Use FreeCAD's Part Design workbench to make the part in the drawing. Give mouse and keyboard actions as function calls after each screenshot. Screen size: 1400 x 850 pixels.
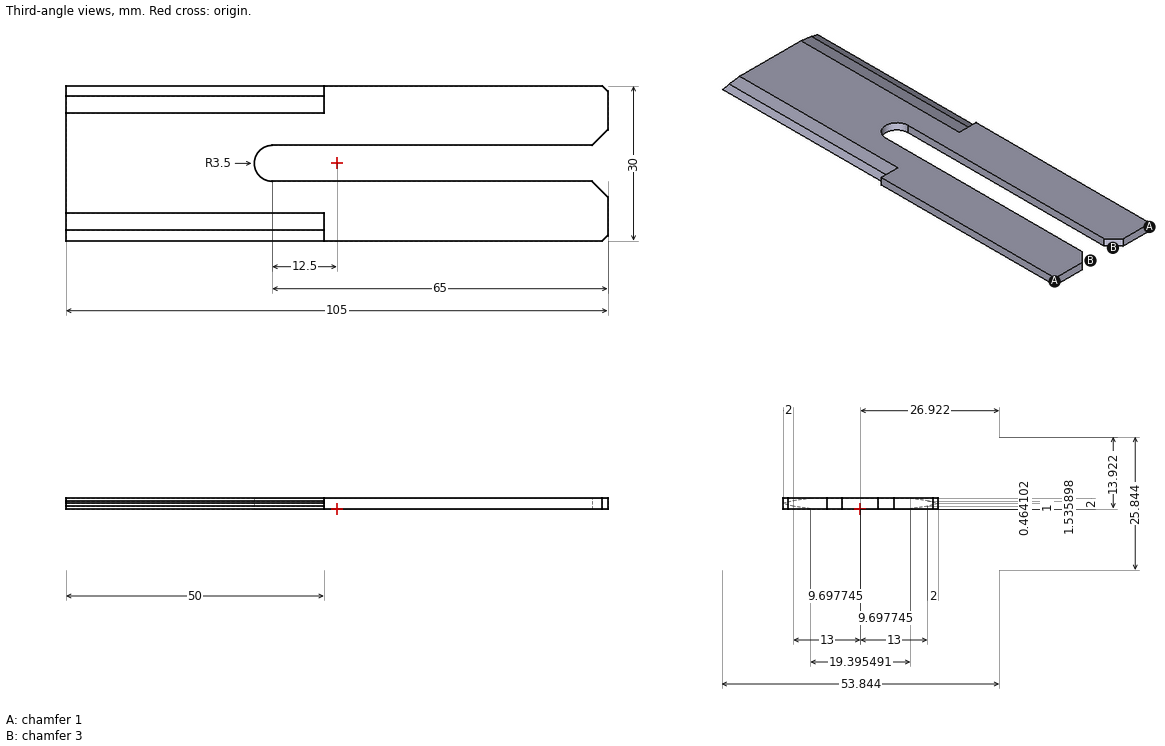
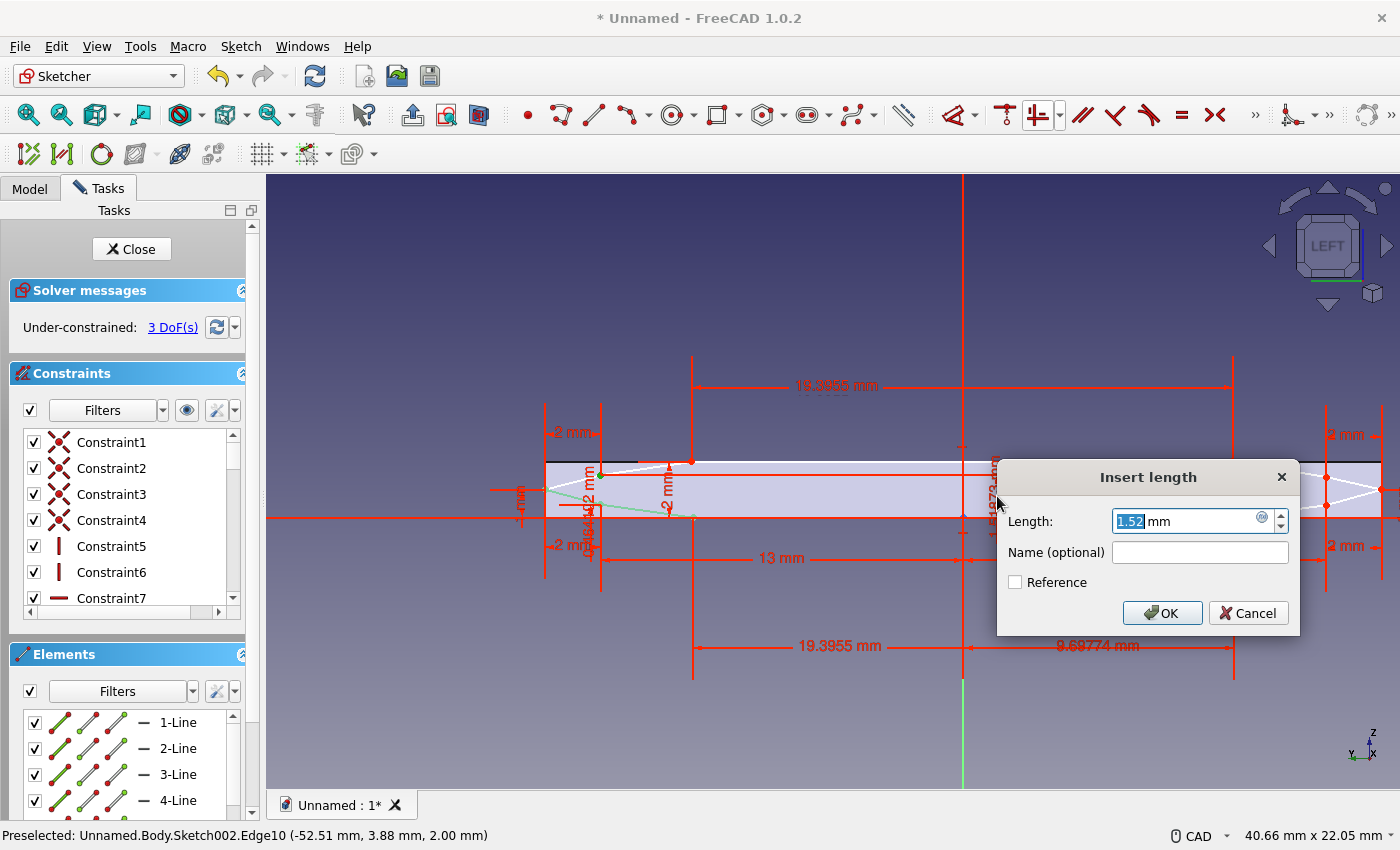
text(1.535898)
key(Return)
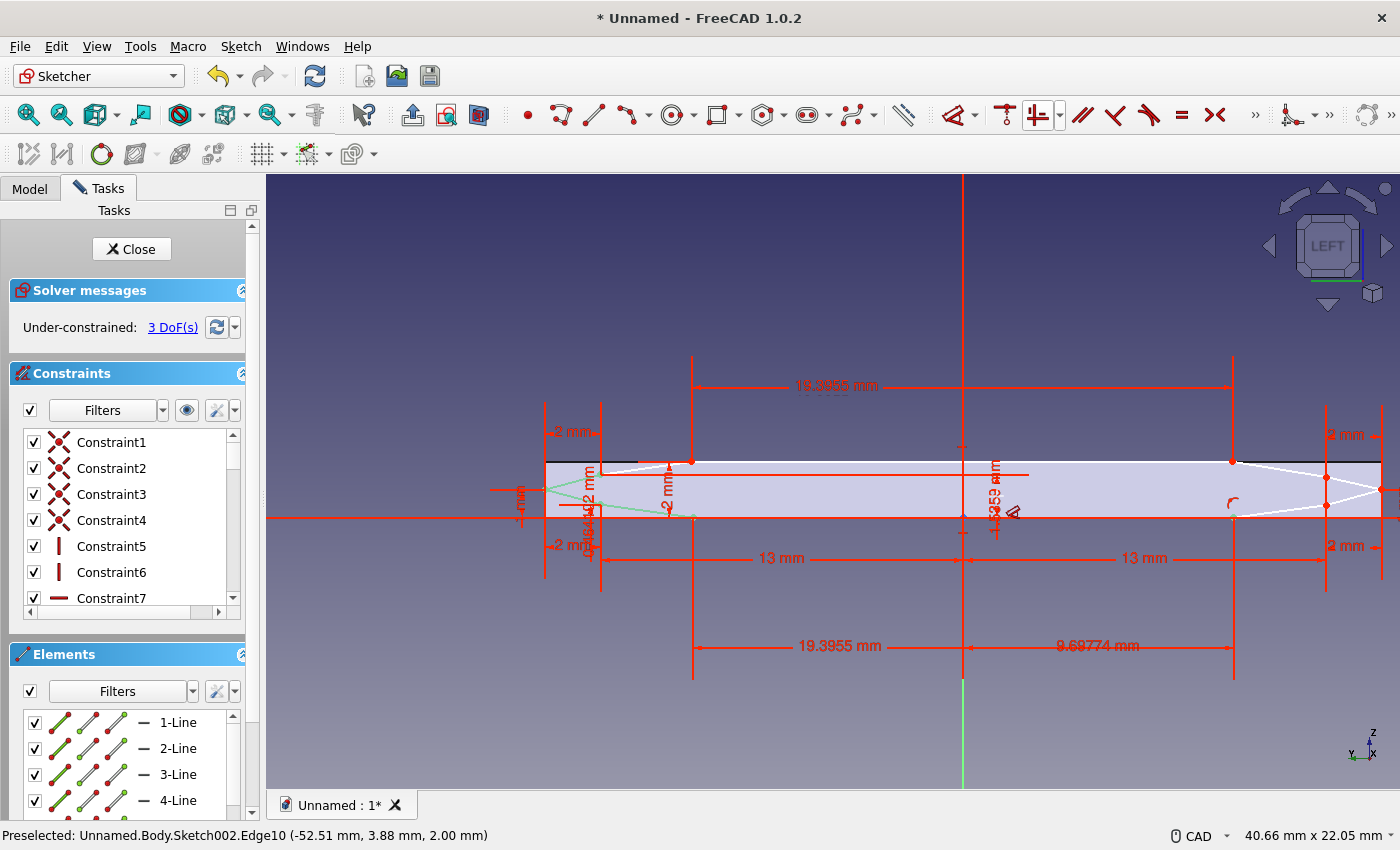
click(692, 462)
click(890, 552)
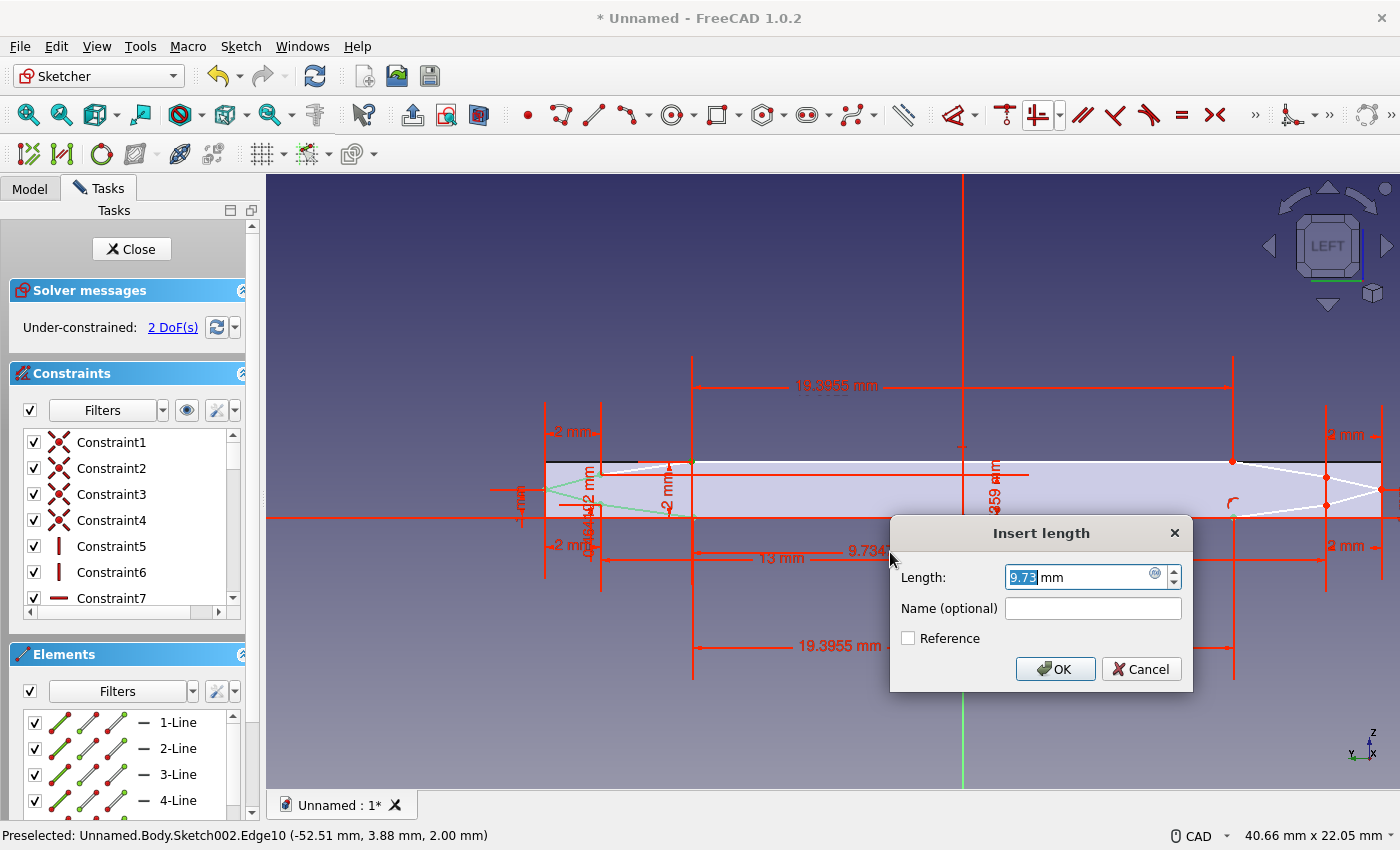
text(9.697745)
key(Return)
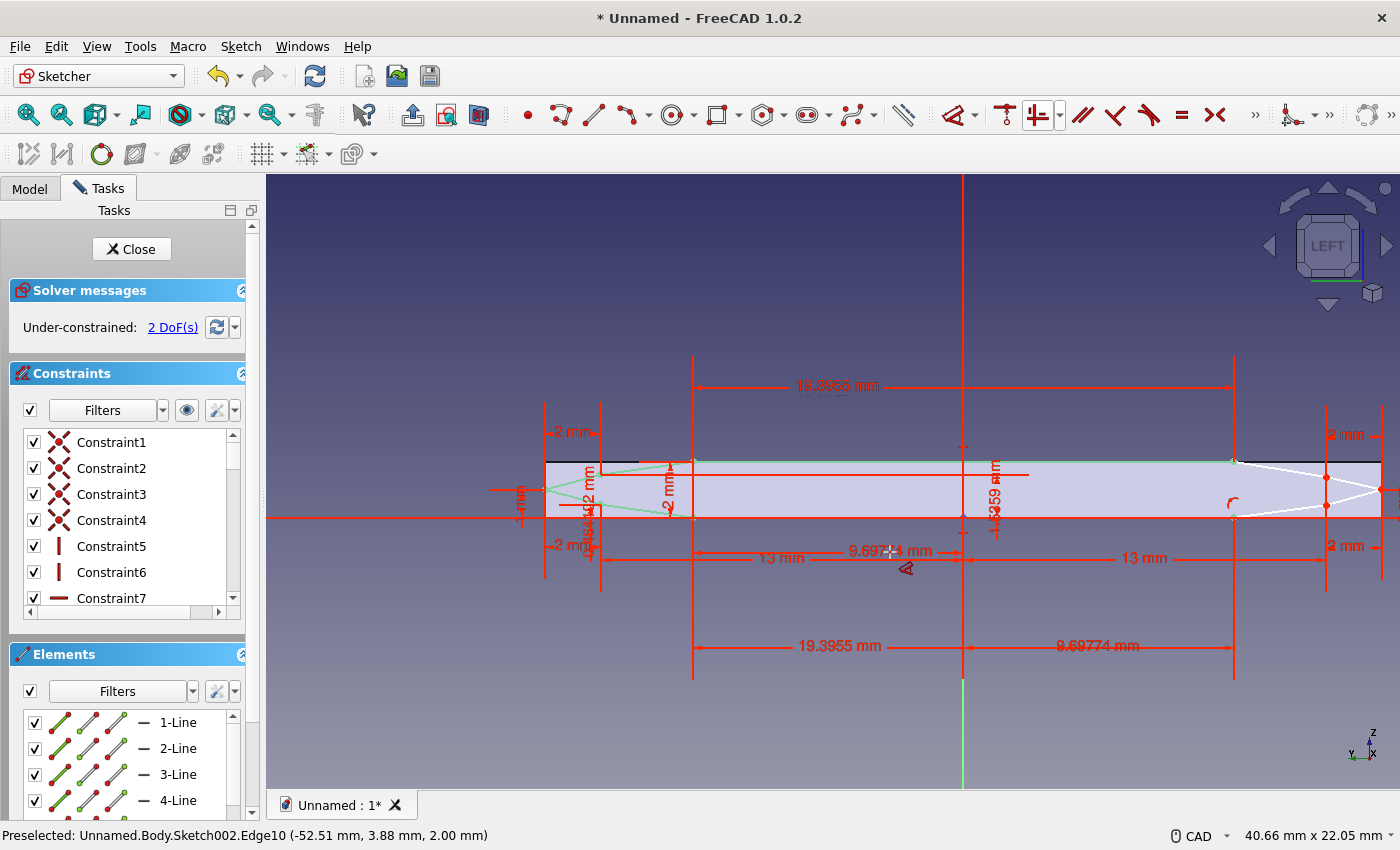
scroll(602, 475, down, 4)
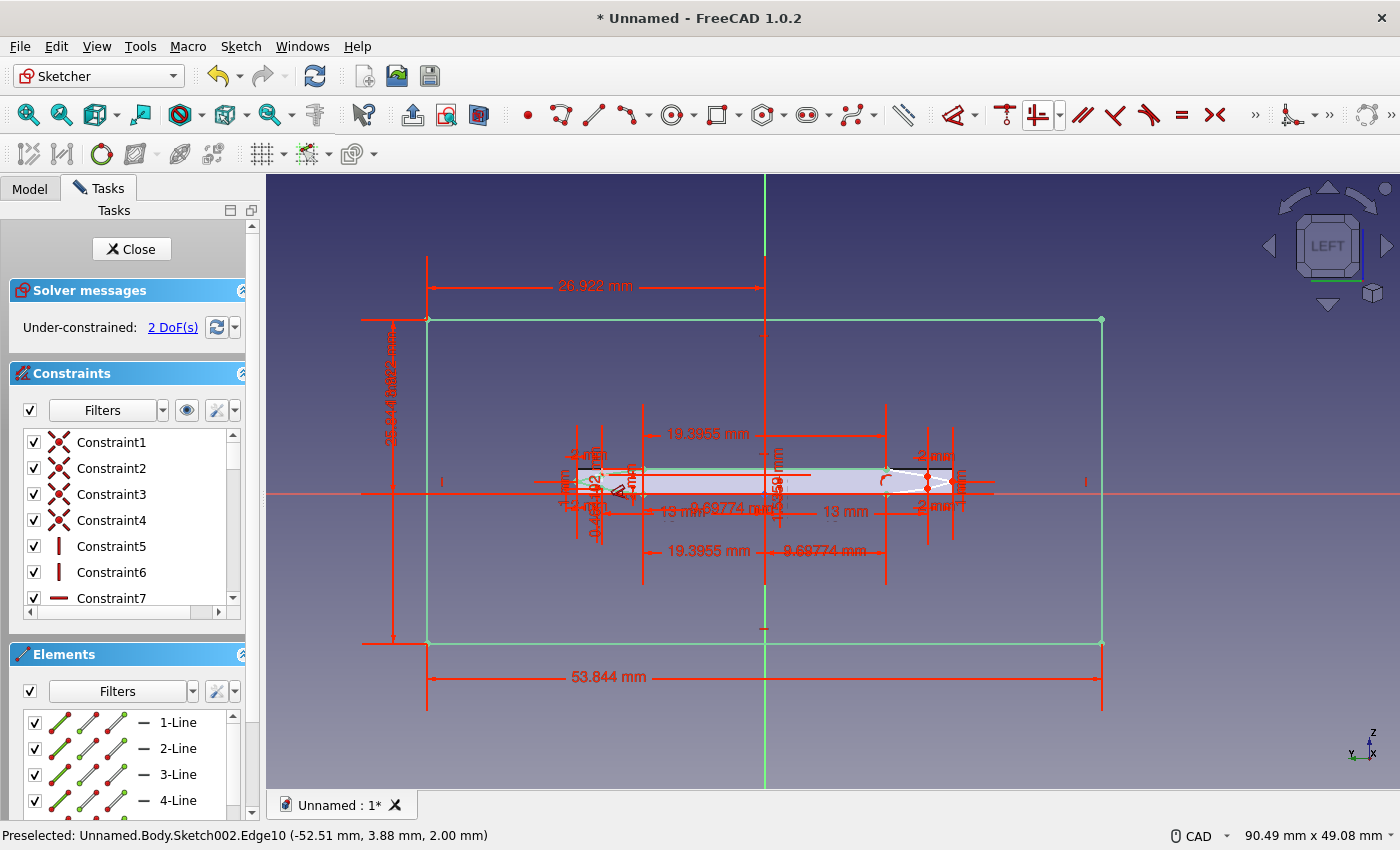
scroll(928, 476, up, 4)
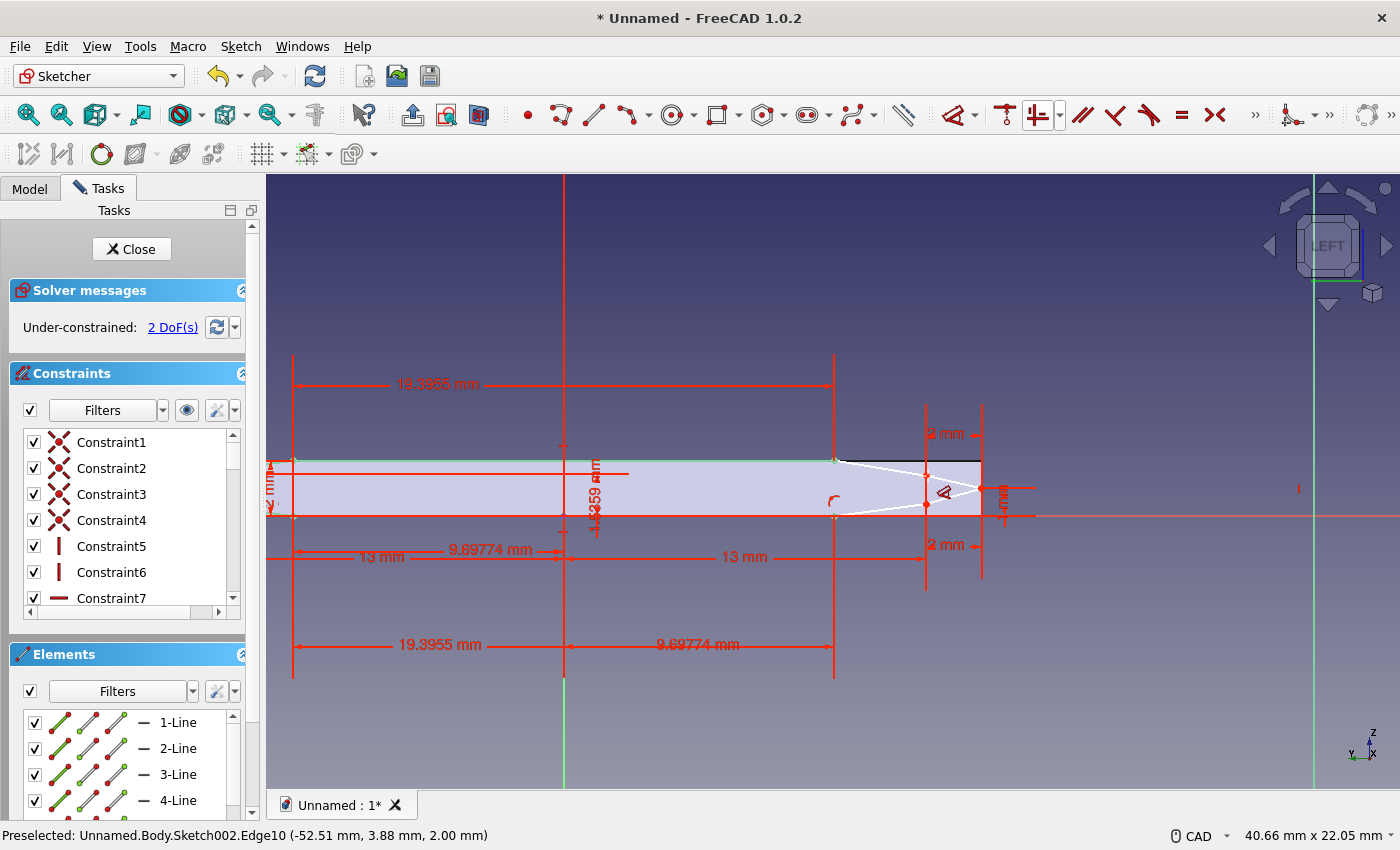
click(926, 476)
click(506, 496)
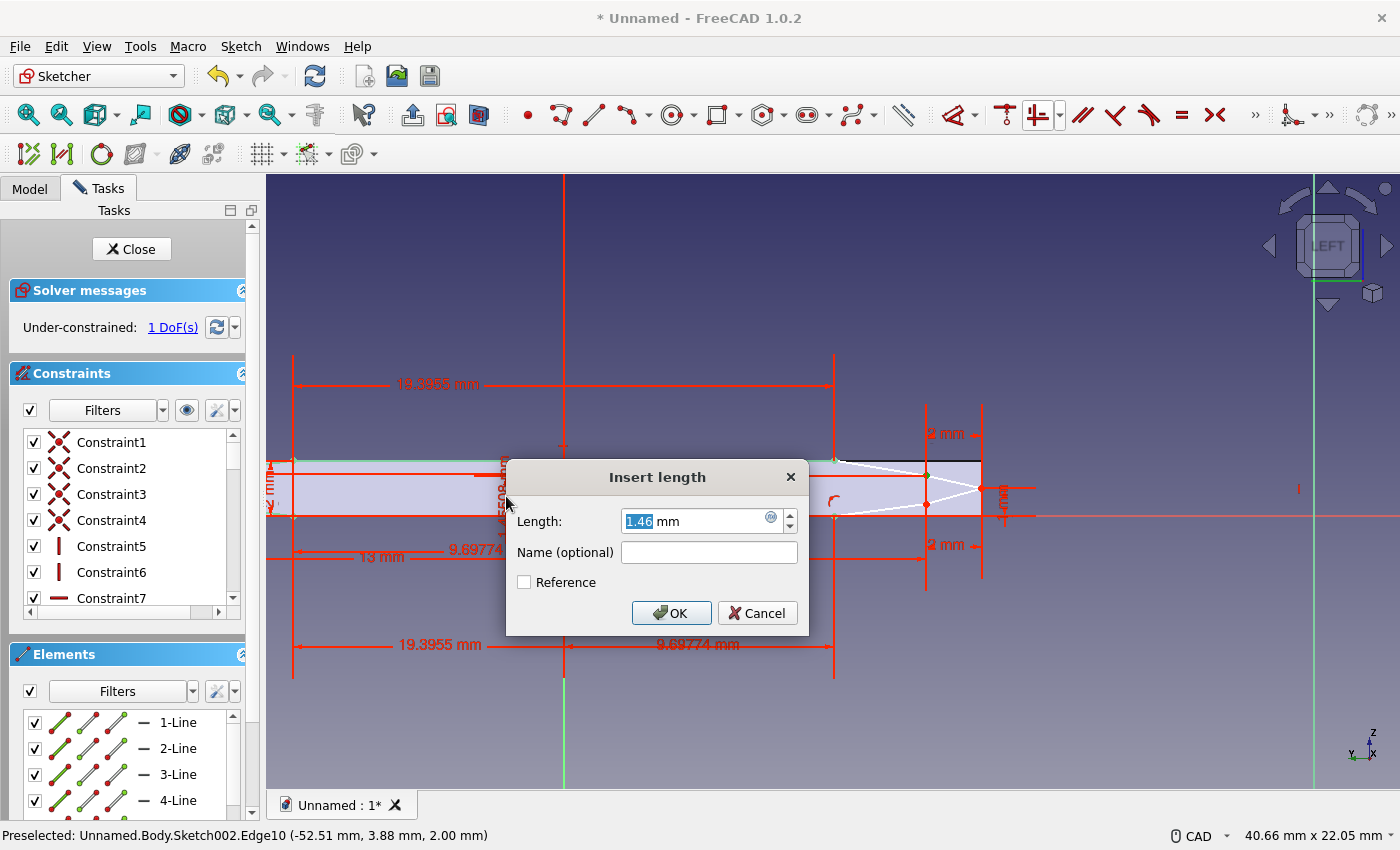
text(1.535898)
key(Return)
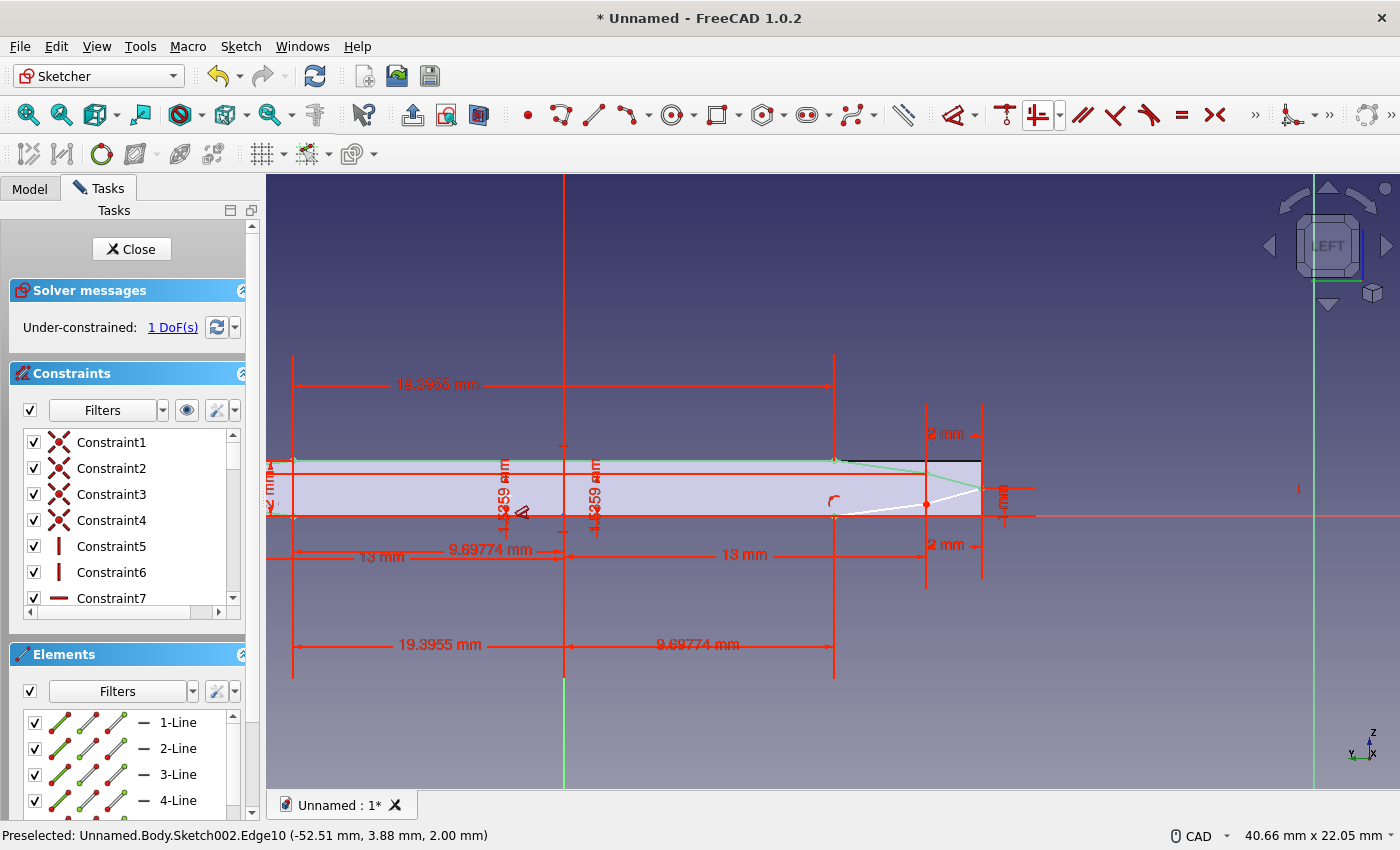
scroll(926, 504, up, 6)